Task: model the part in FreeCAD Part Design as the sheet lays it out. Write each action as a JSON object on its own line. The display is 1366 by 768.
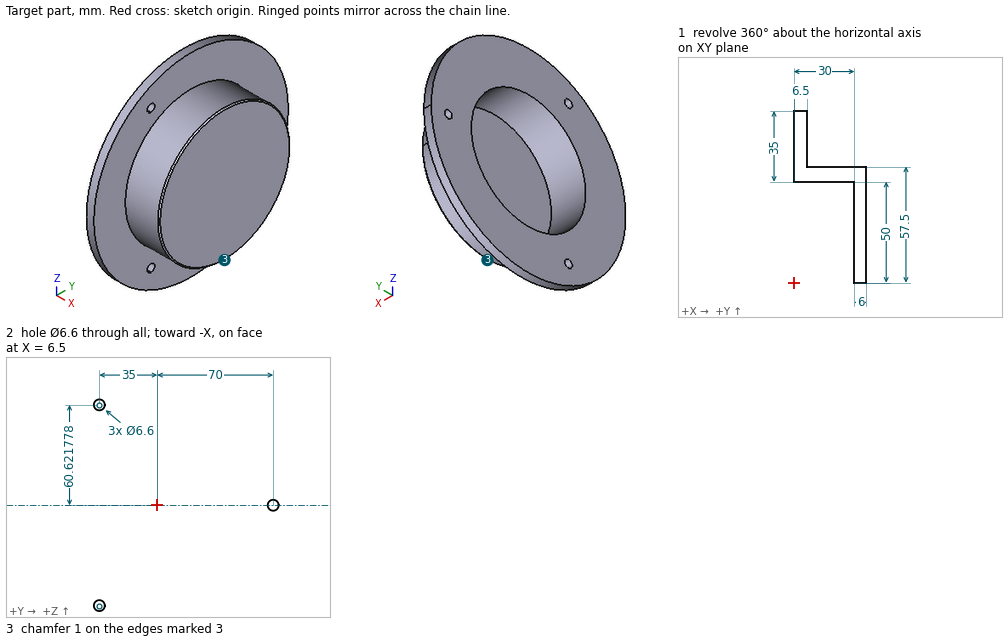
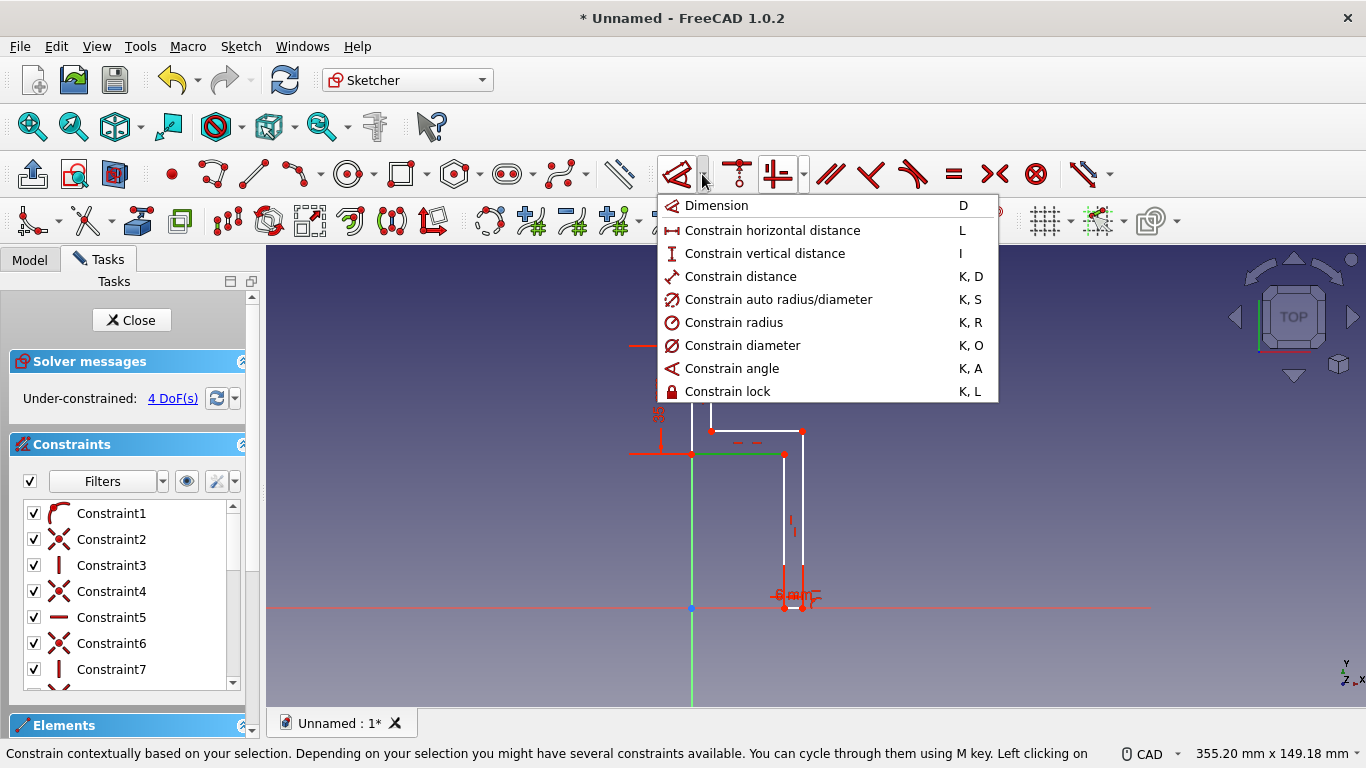
{"action": "left_click", "coordinate": [828, 230]}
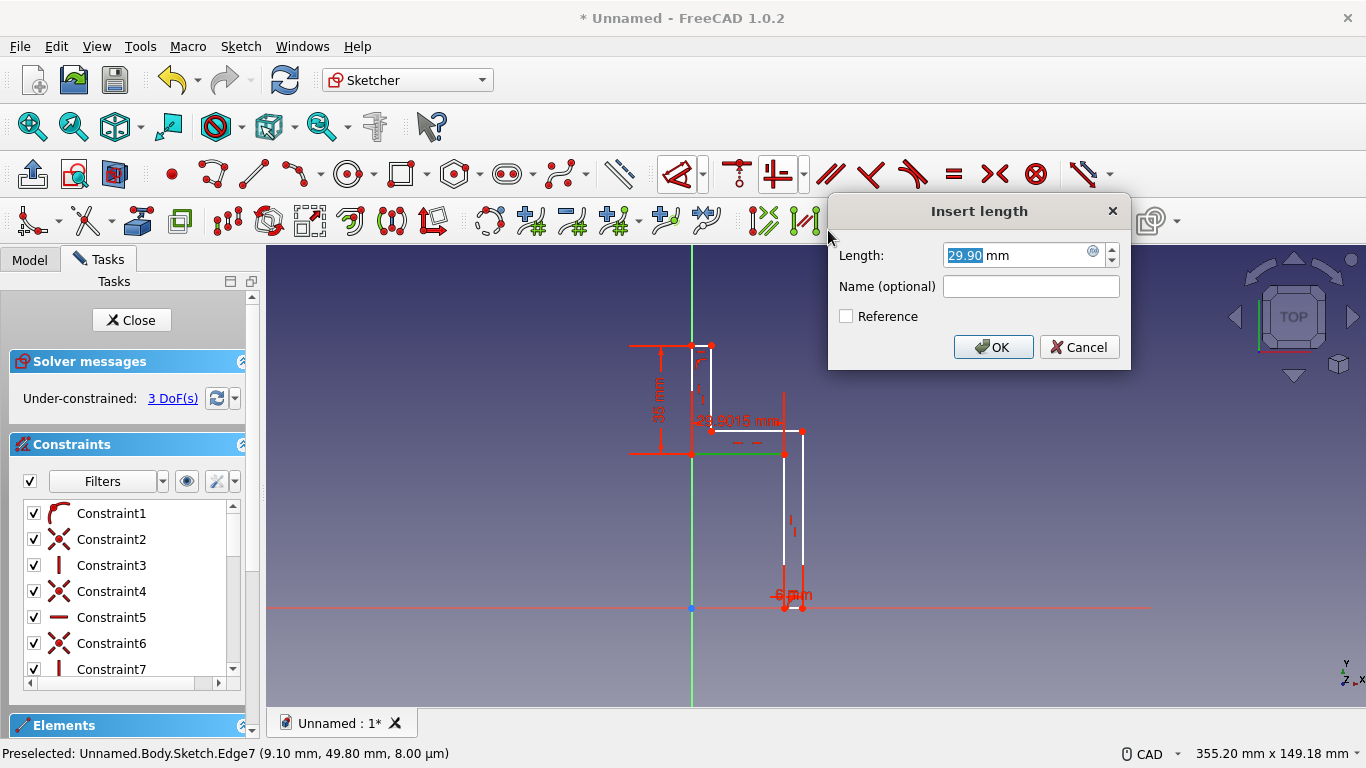
{"action": "type", "text": "30"}
{"action": "key", "text": "Return"}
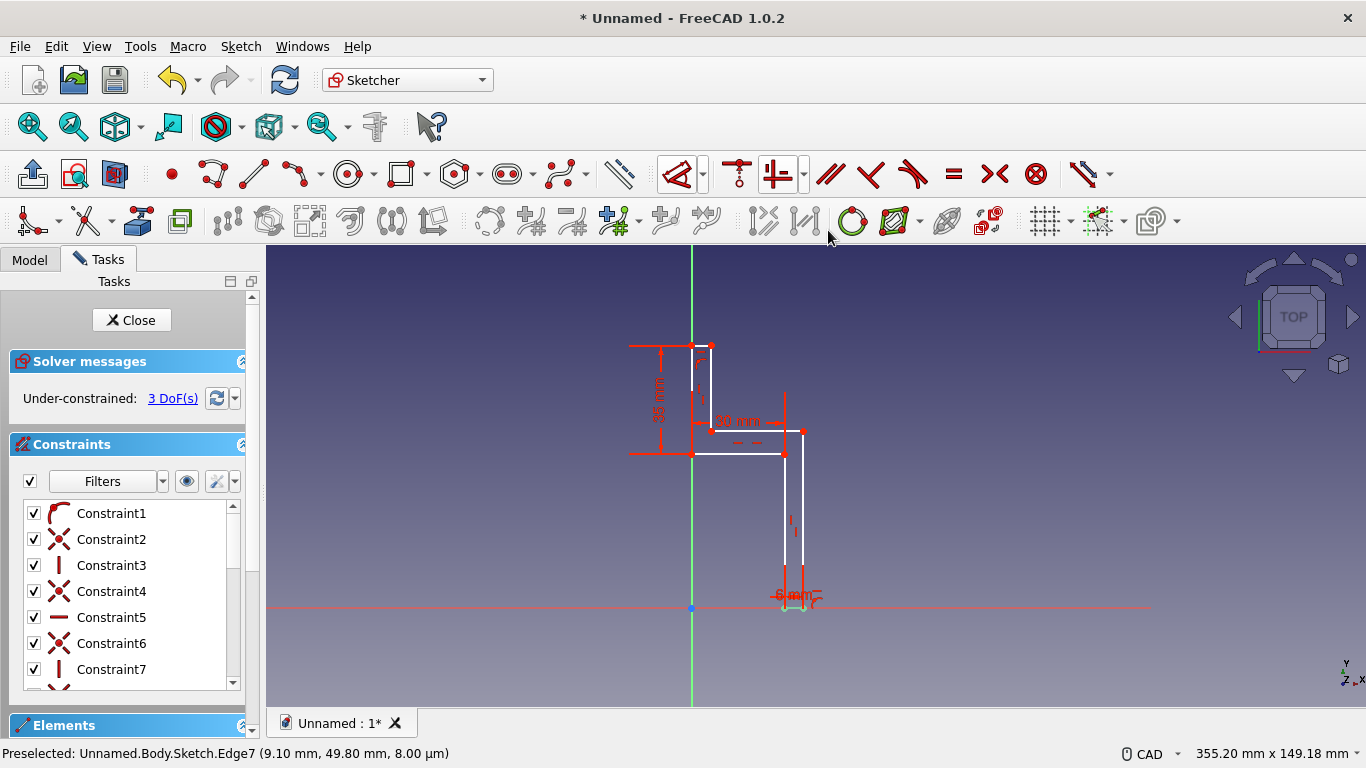
{"action": "left_click", "coordinate": [785, 500]}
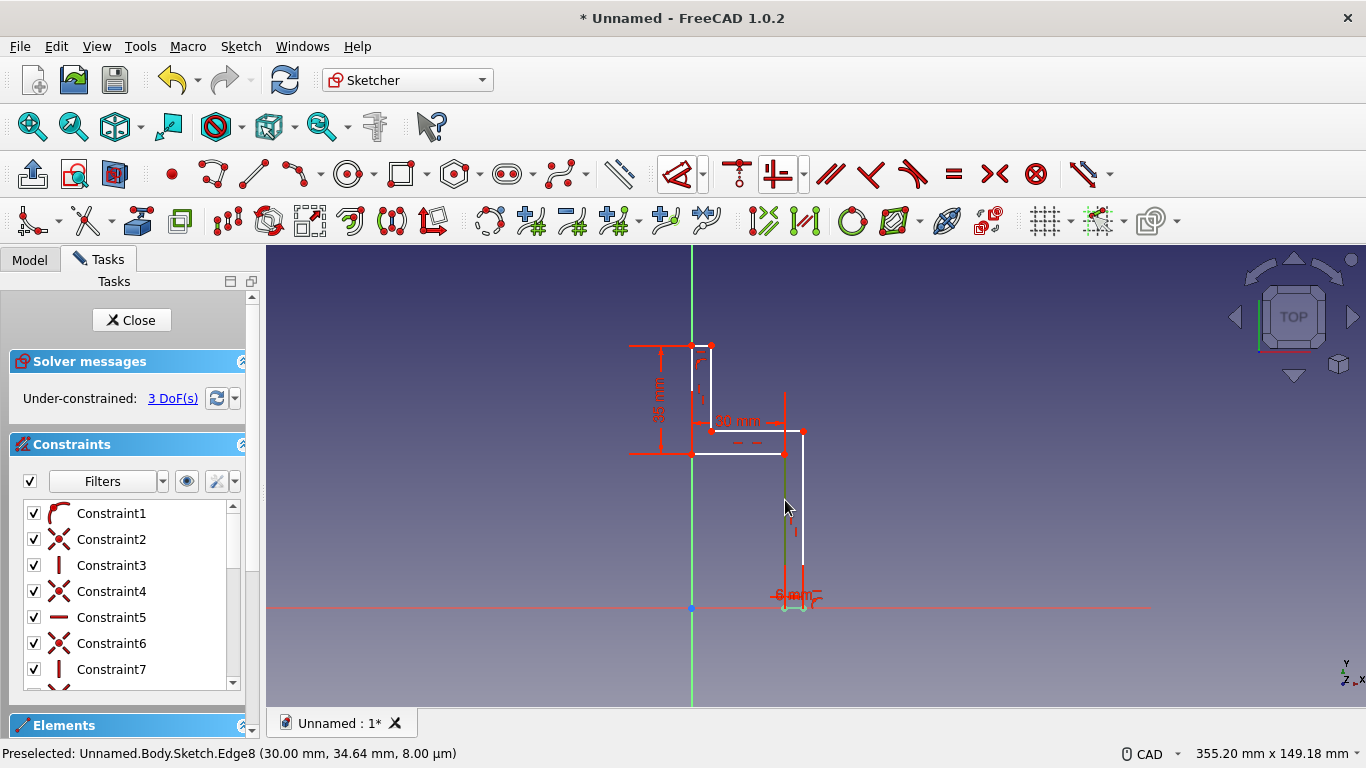
{"action": "key", "text": "i"}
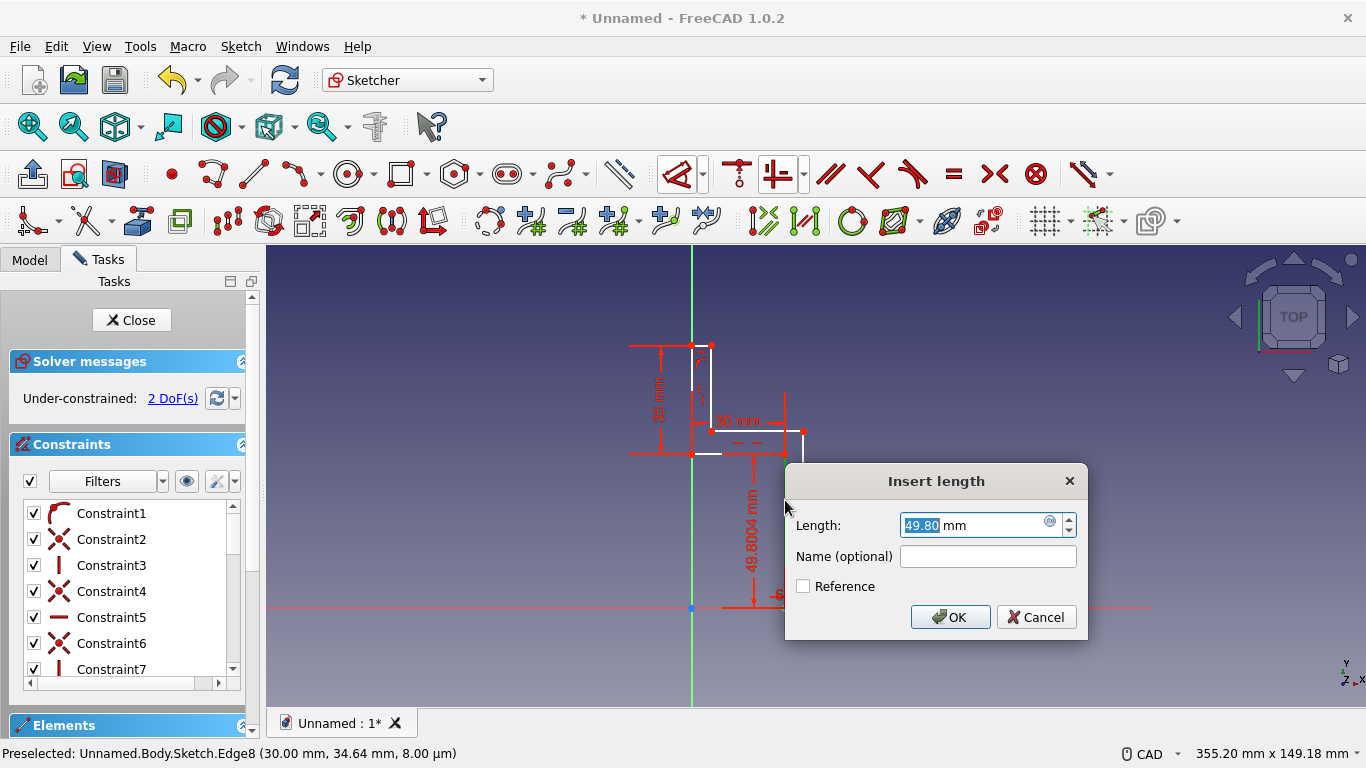
{"action": "type", "text": "50"}
{"action": "key", "text": "Return"}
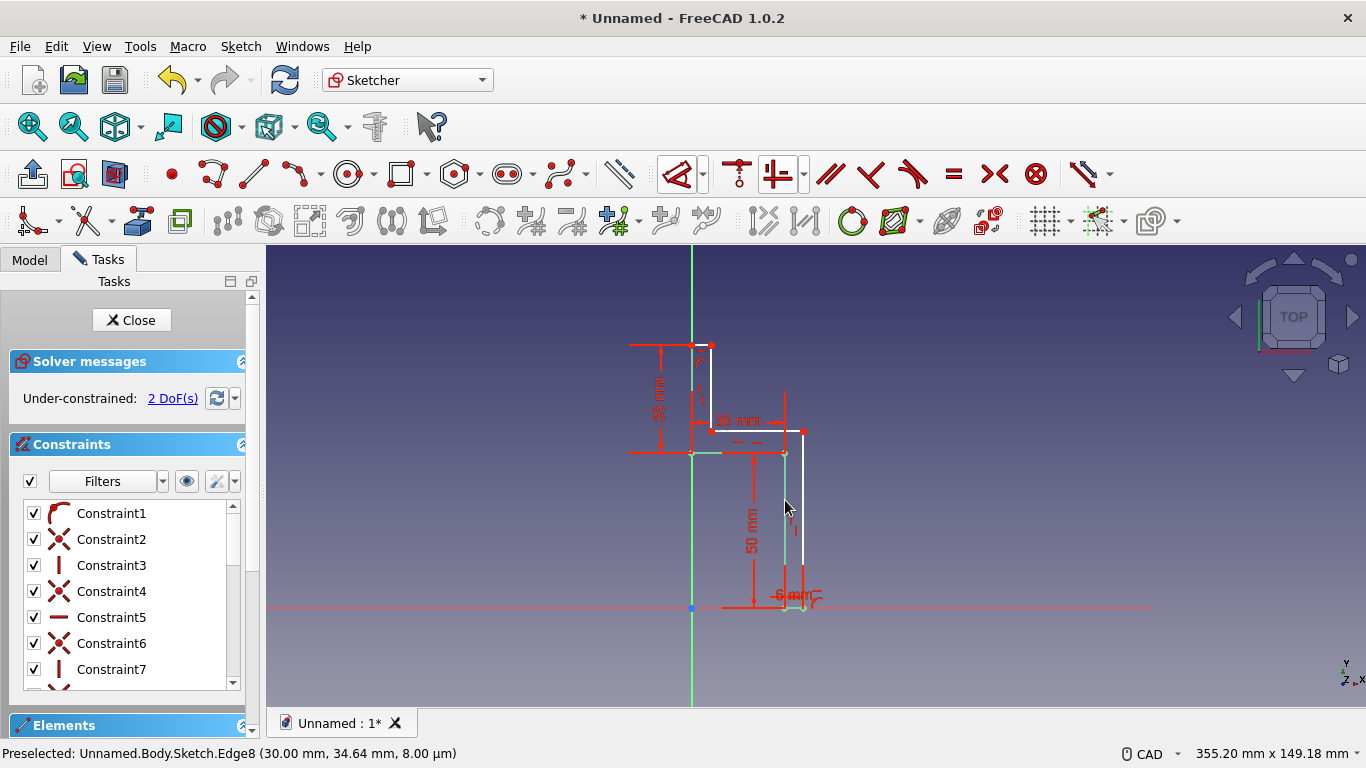
{"action": "scroll", "coordinate": [702, 345], "scroll_direction": "up", "scroll_amount": 4}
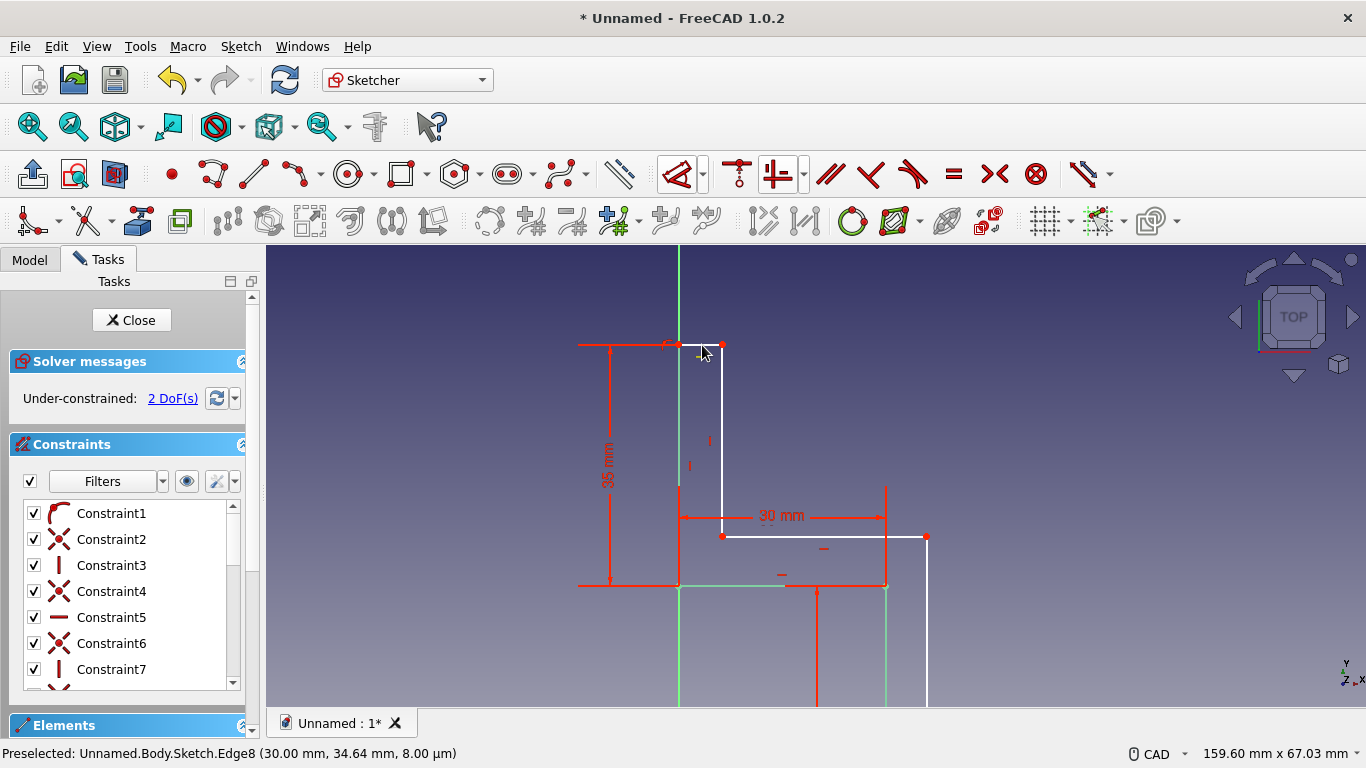
{"action": "left_click", "coordinate": [701, 345]}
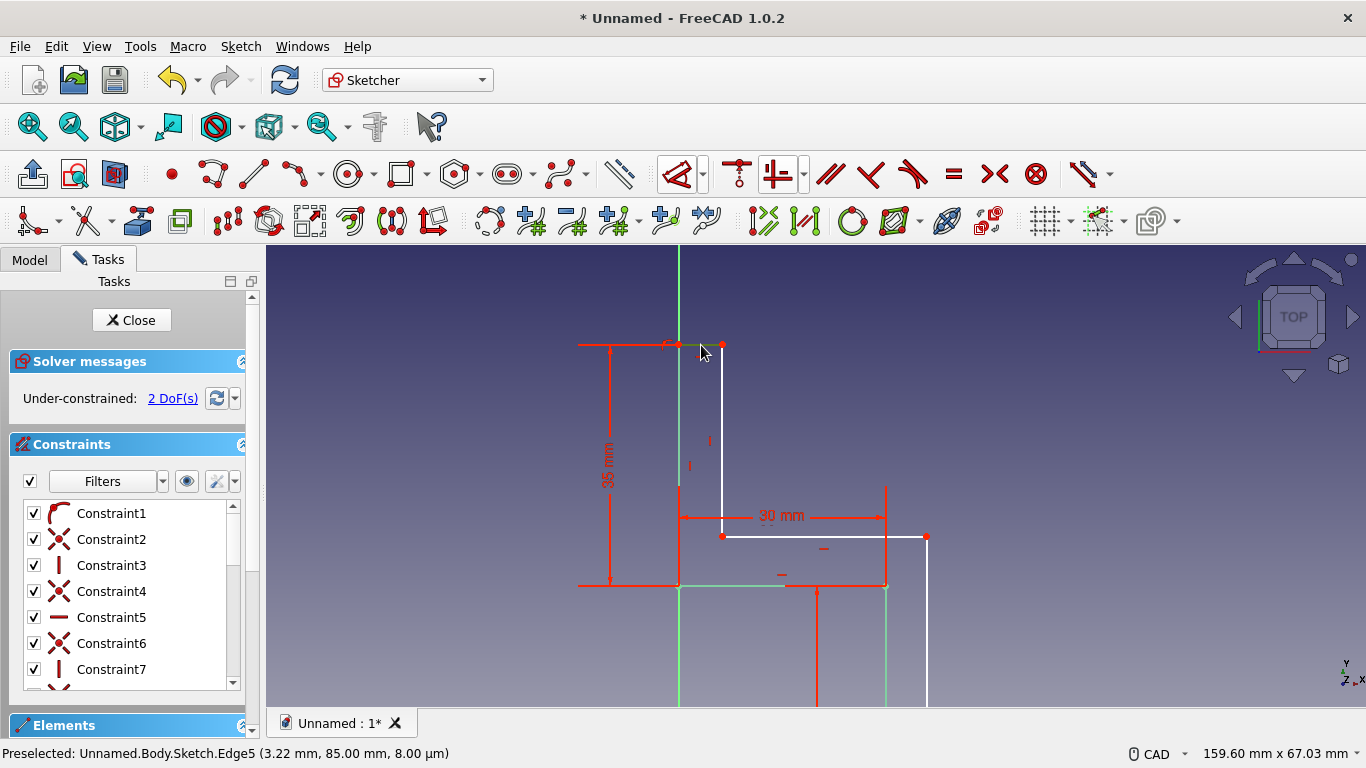
{"action": "key", "text": "l"}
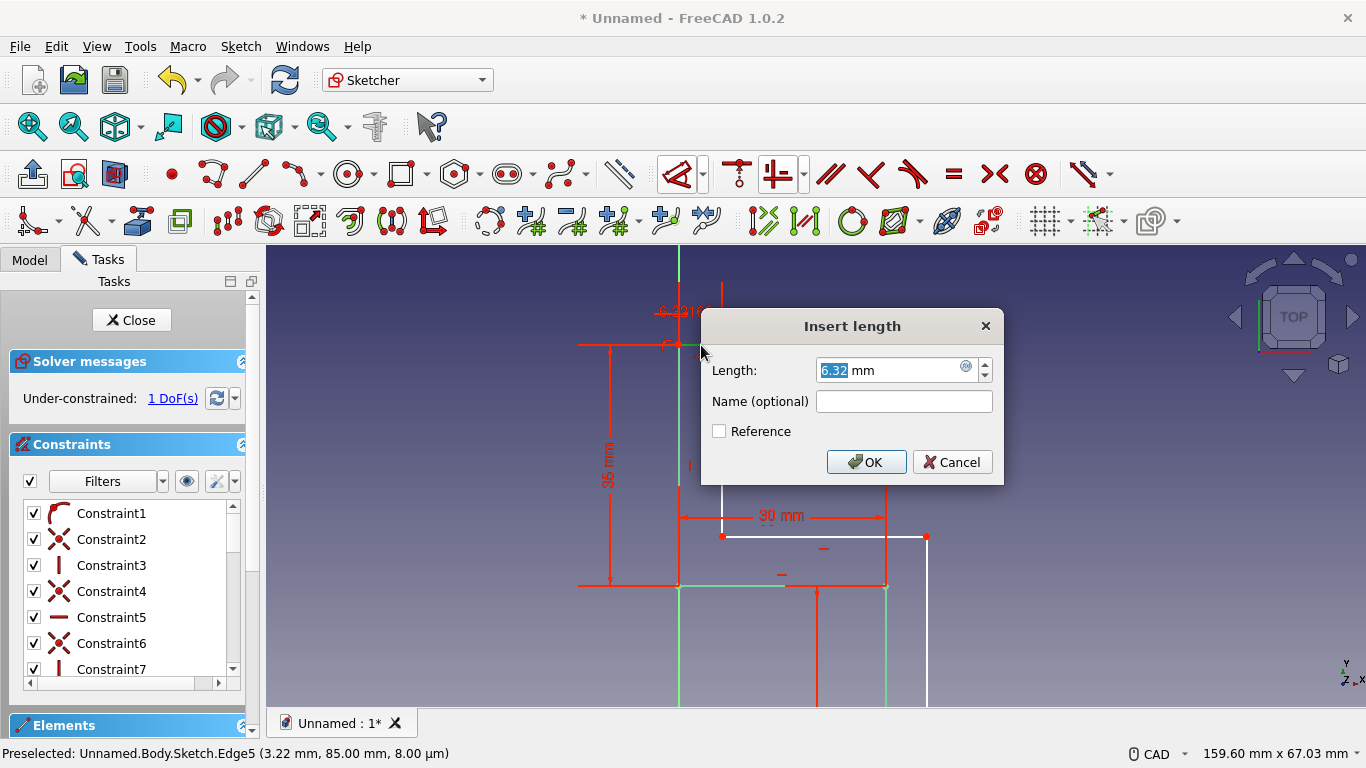
{"action": "type", "text": "6.5"}
{"action": "key", "text": "Return"}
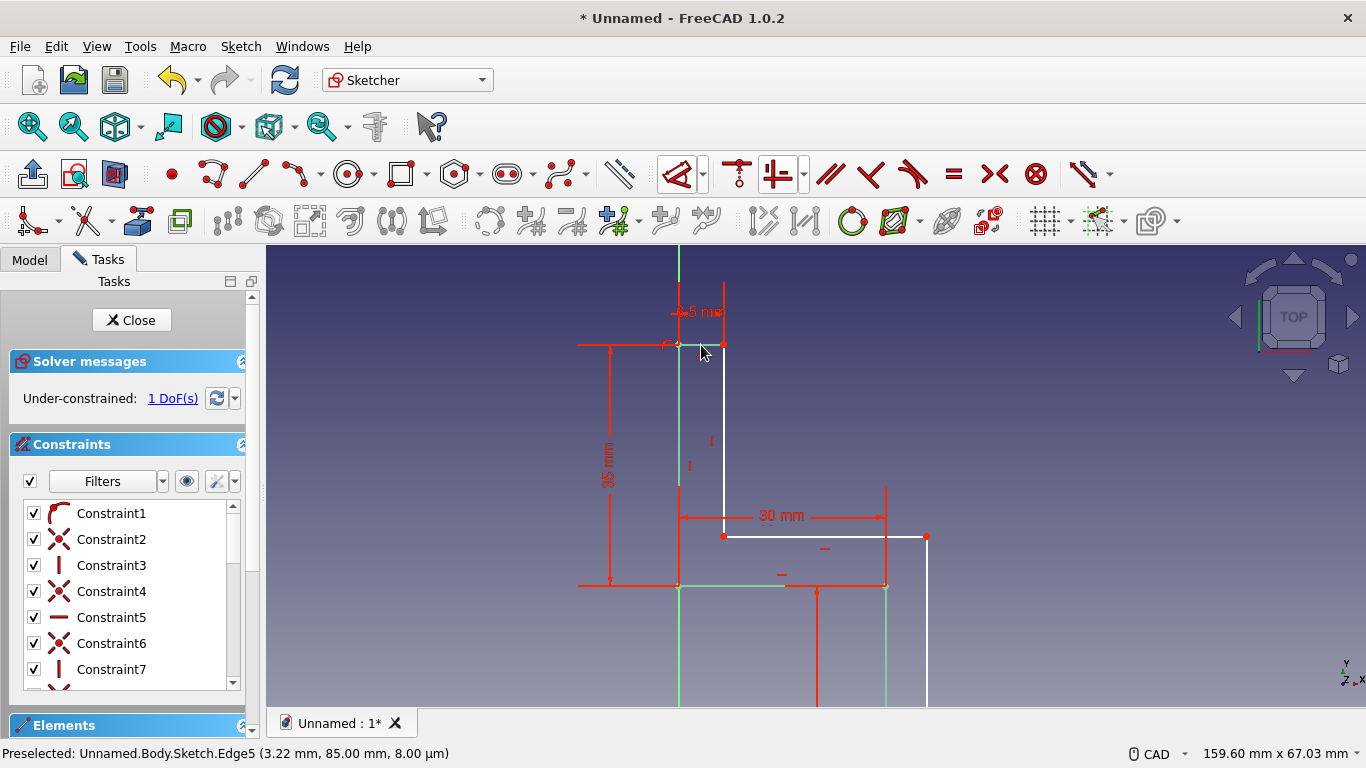
{"action": "left_click", "coordinate": [927, 655]}